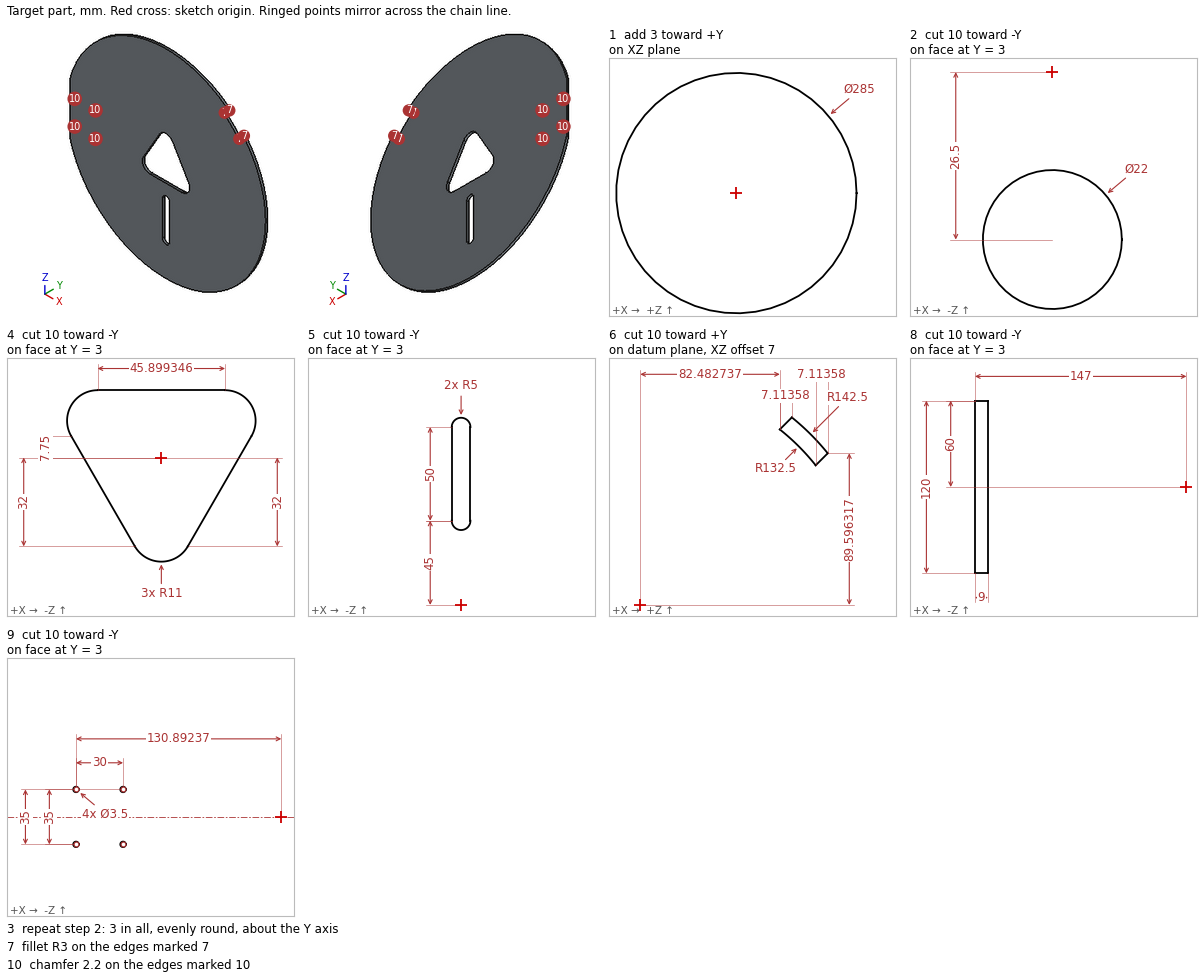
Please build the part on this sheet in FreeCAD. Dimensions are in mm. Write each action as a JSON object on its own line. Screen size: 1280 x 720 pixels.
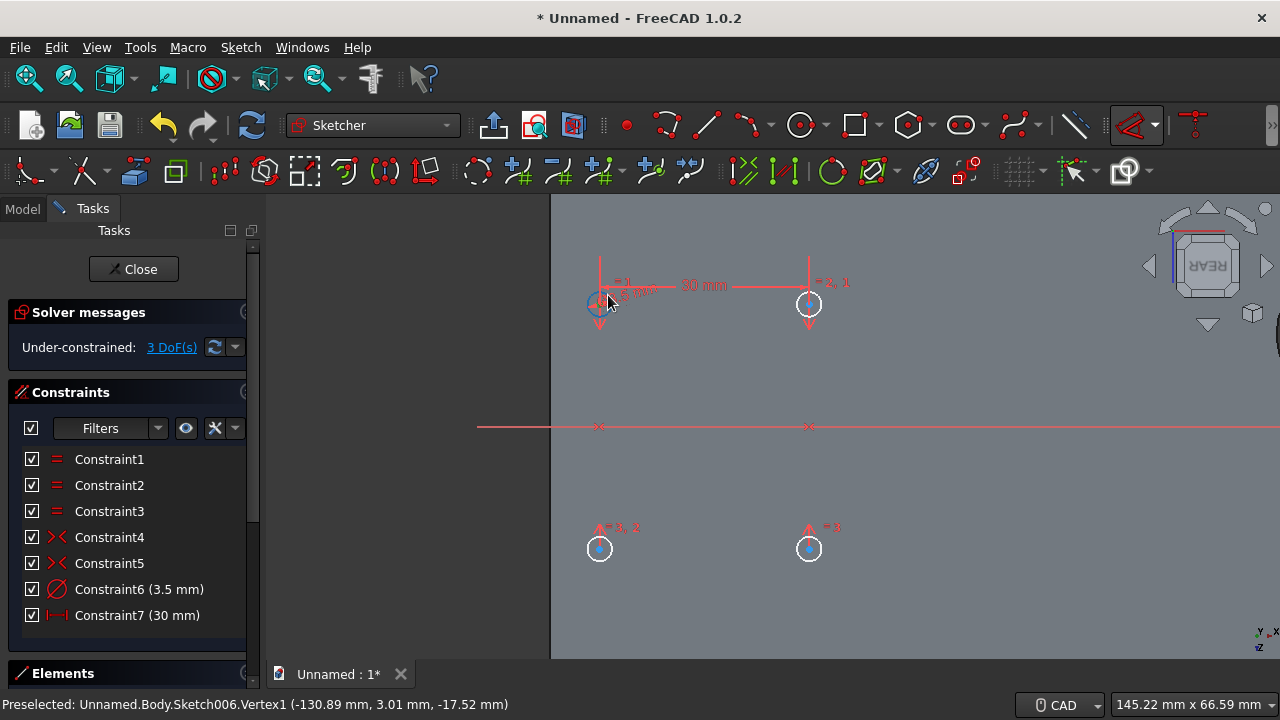
{"action": "left_click", "coordinate": [600, 549]}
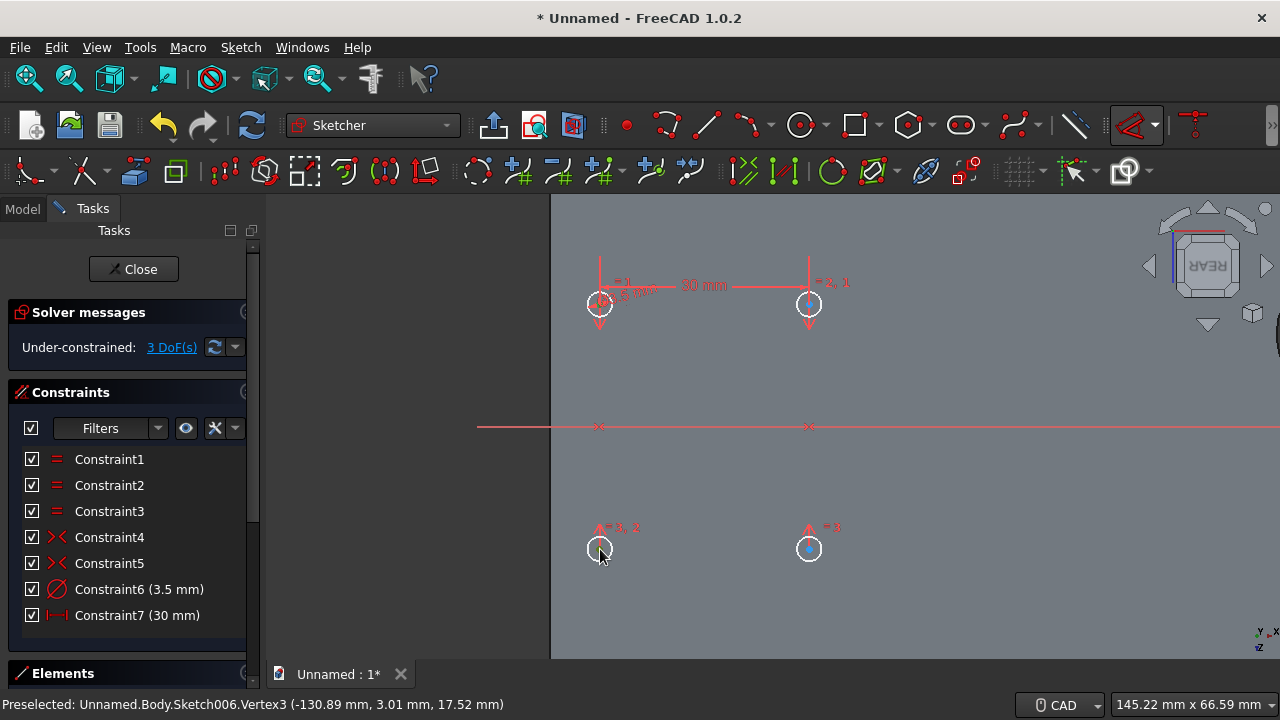
{"action": "key", "text": "i"}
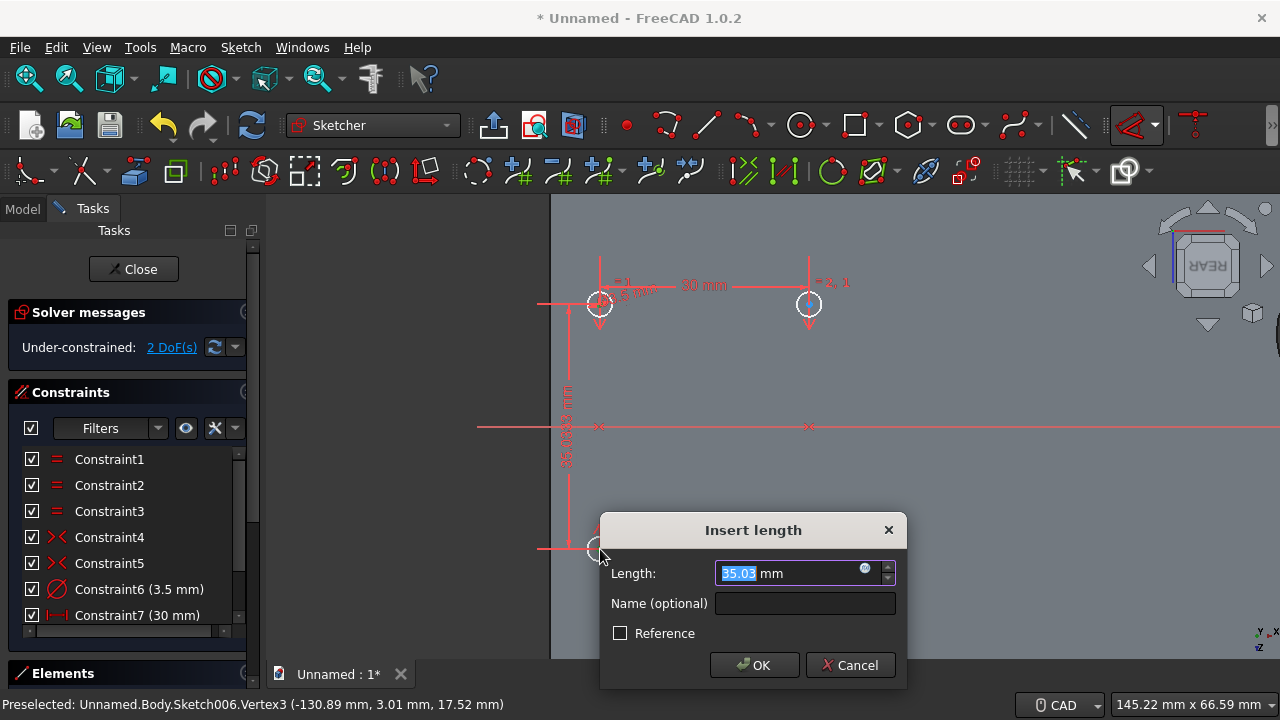
{"action": "type", "text": "35"}
{"action": "key", "text": "Return"}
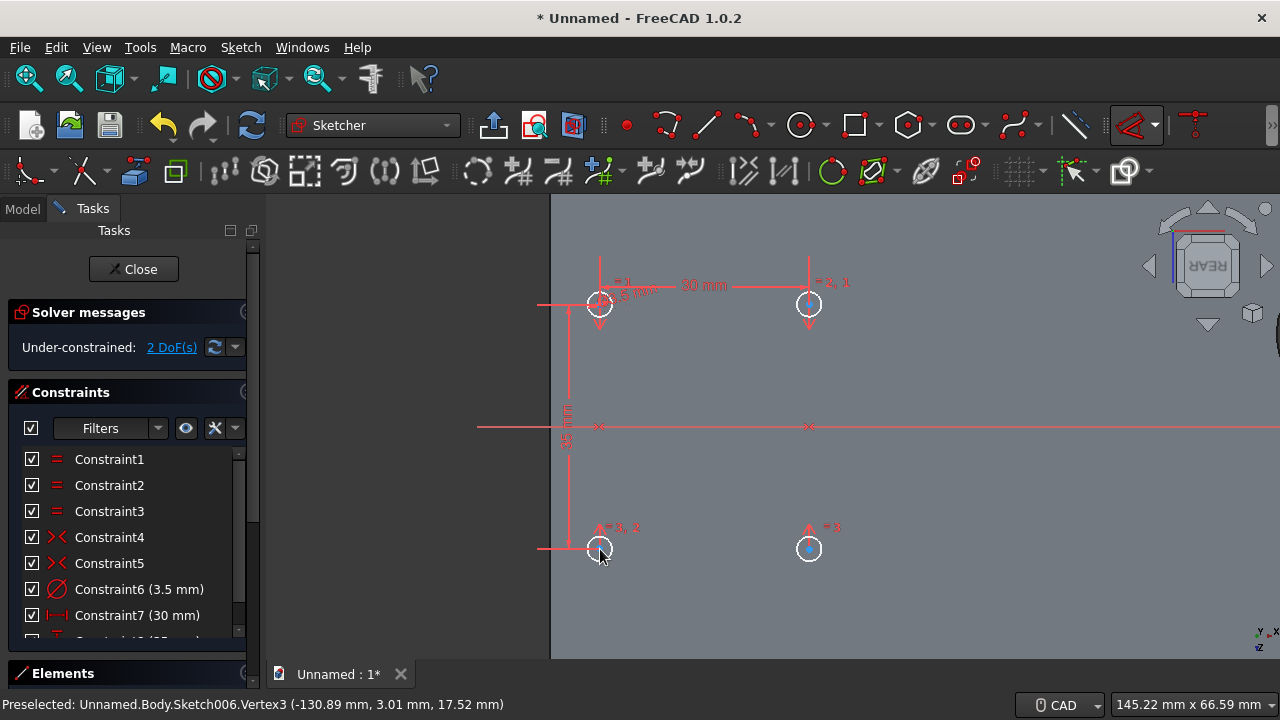
{"action": "left_click", "coordinate": [809, 304]}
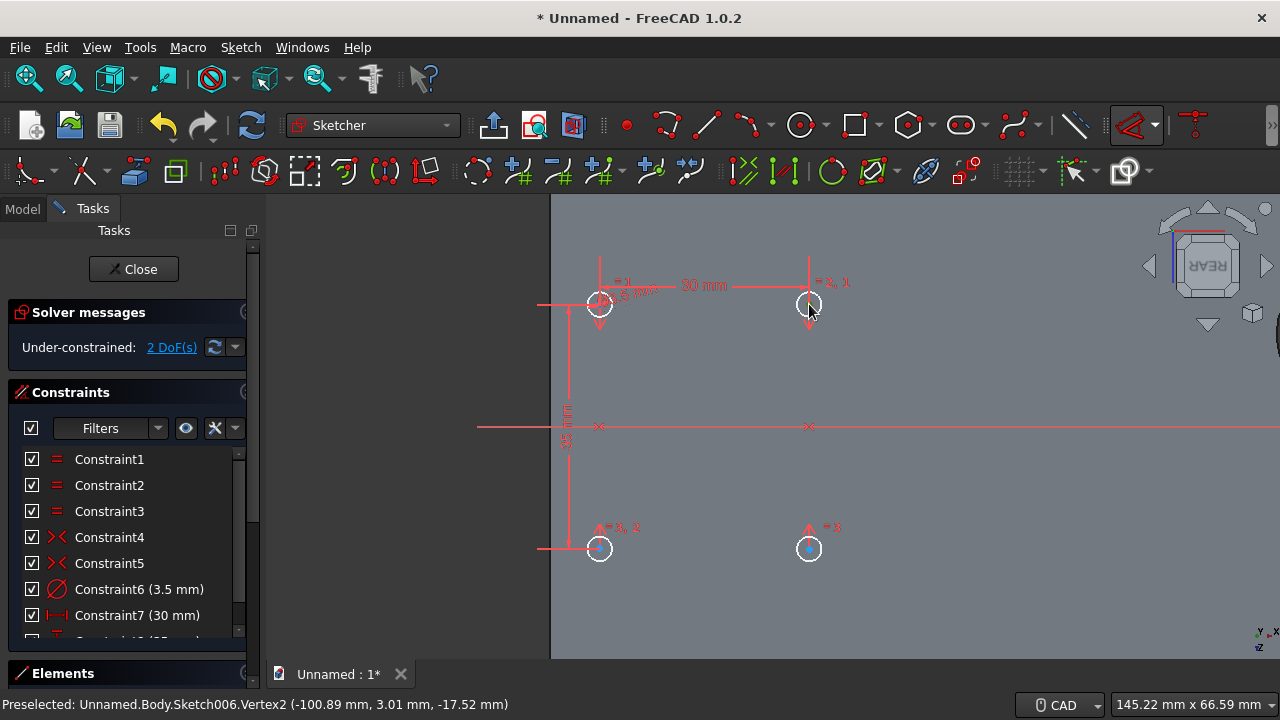
{"action": "left_click", "coordinate": [600, 549]}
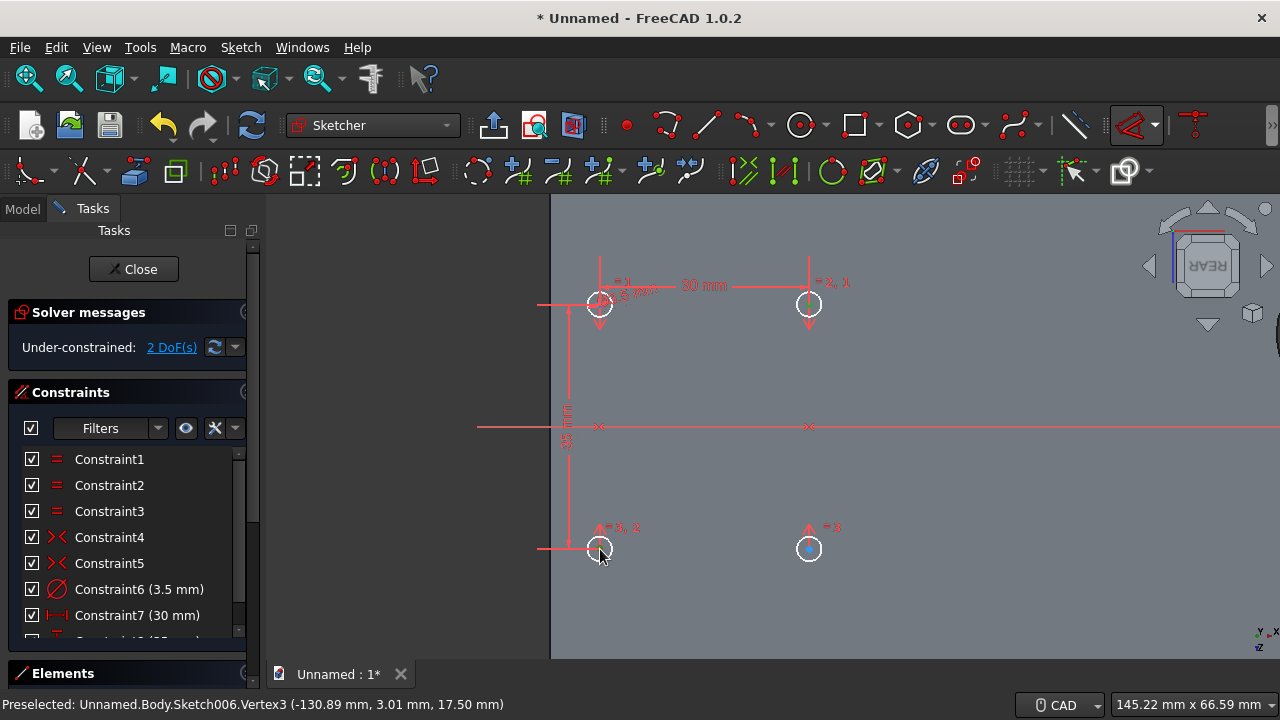
{"action": "key", "text": "i"}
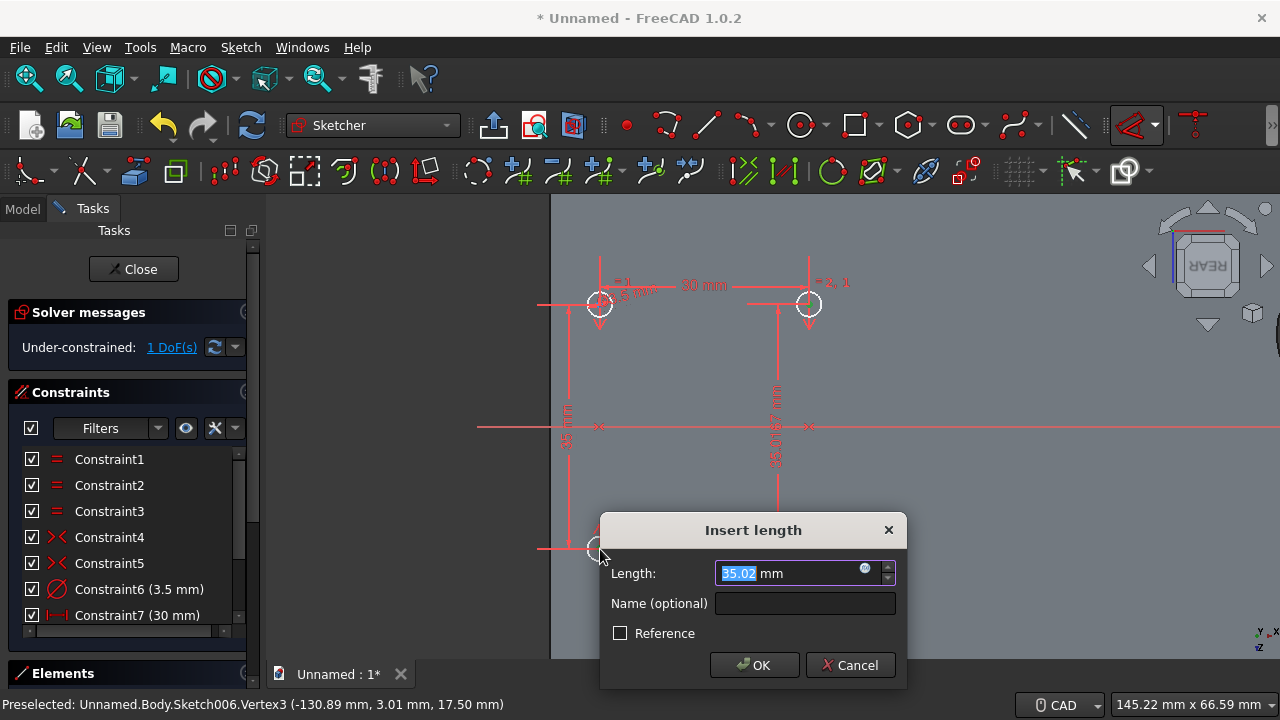
{"action": "type", "text": "35"}
{"action": "key", "text": "Return"}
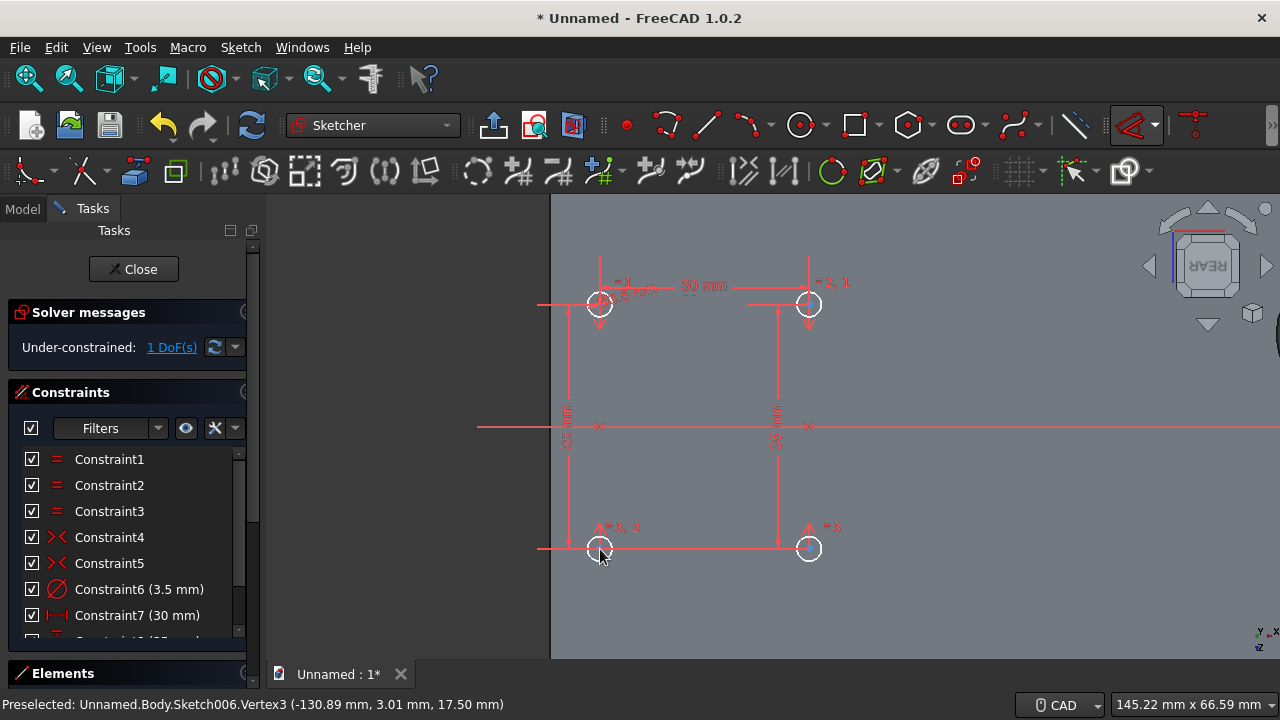
{"action": "left_click", "coordinate": [600, 305]}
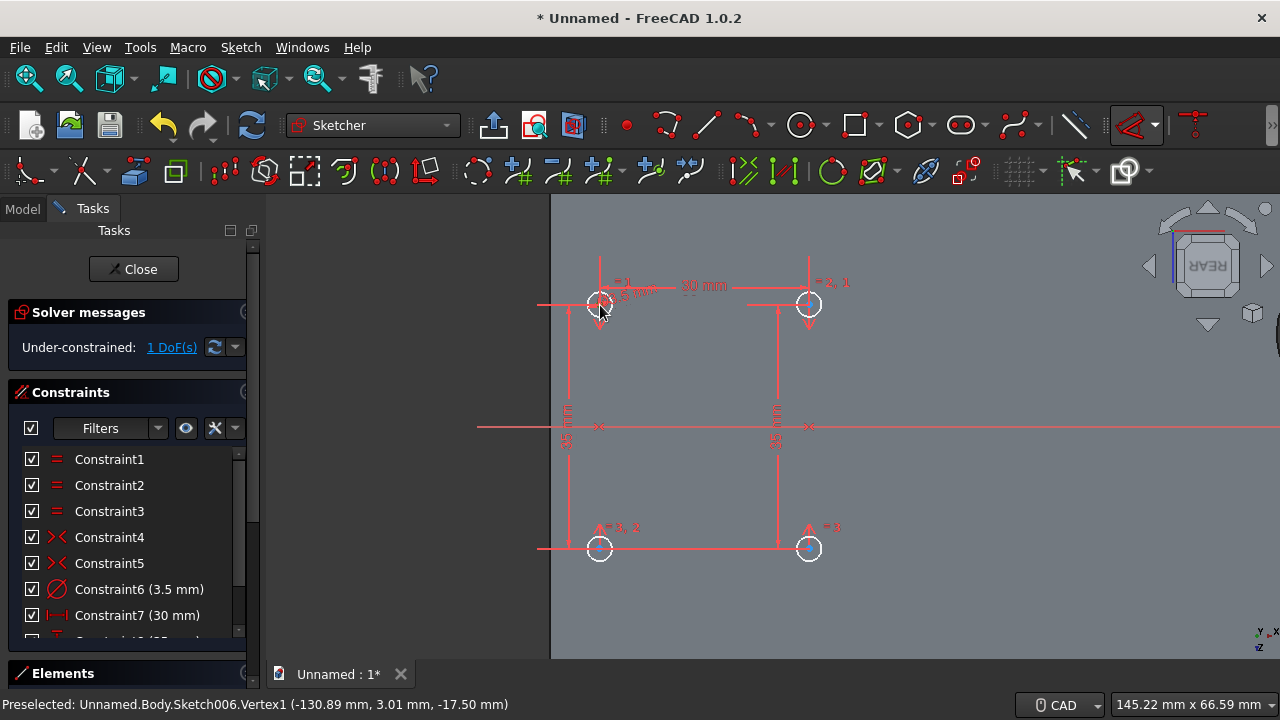
{"action": "left_click", "coordinate": [1158, 126]}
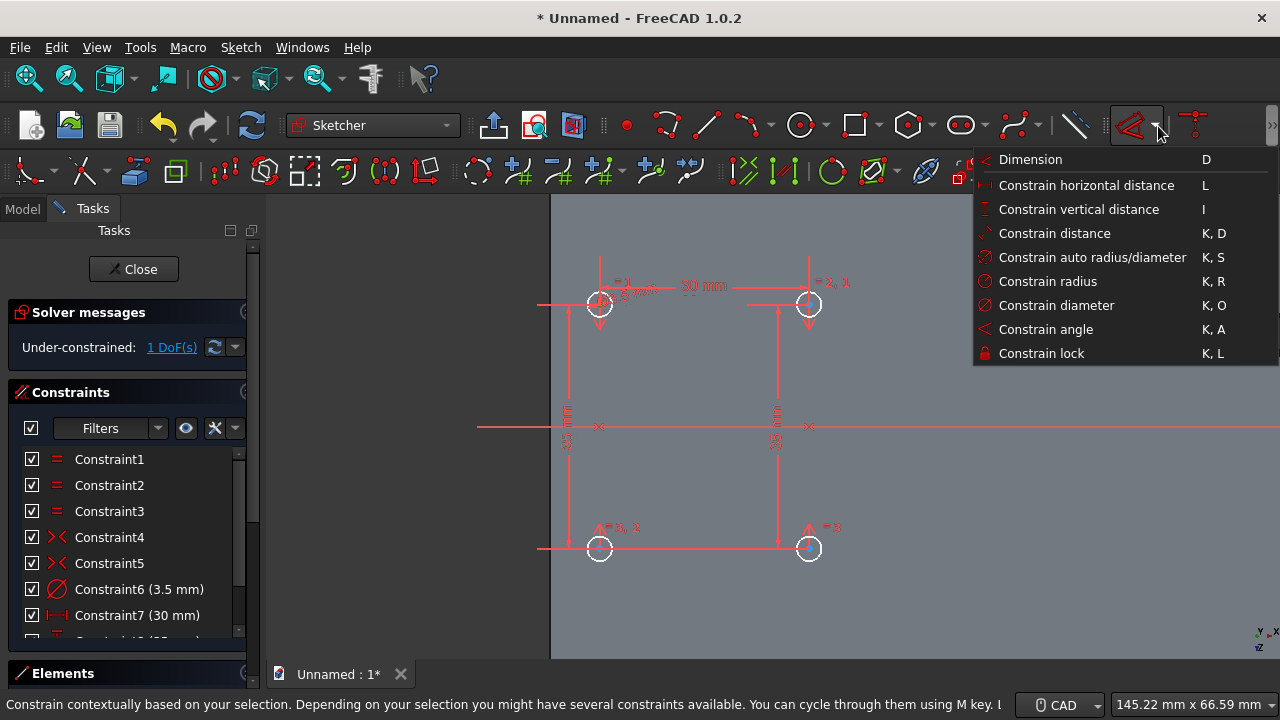
{"action": "left_click", "coordinate": [1126, 185]}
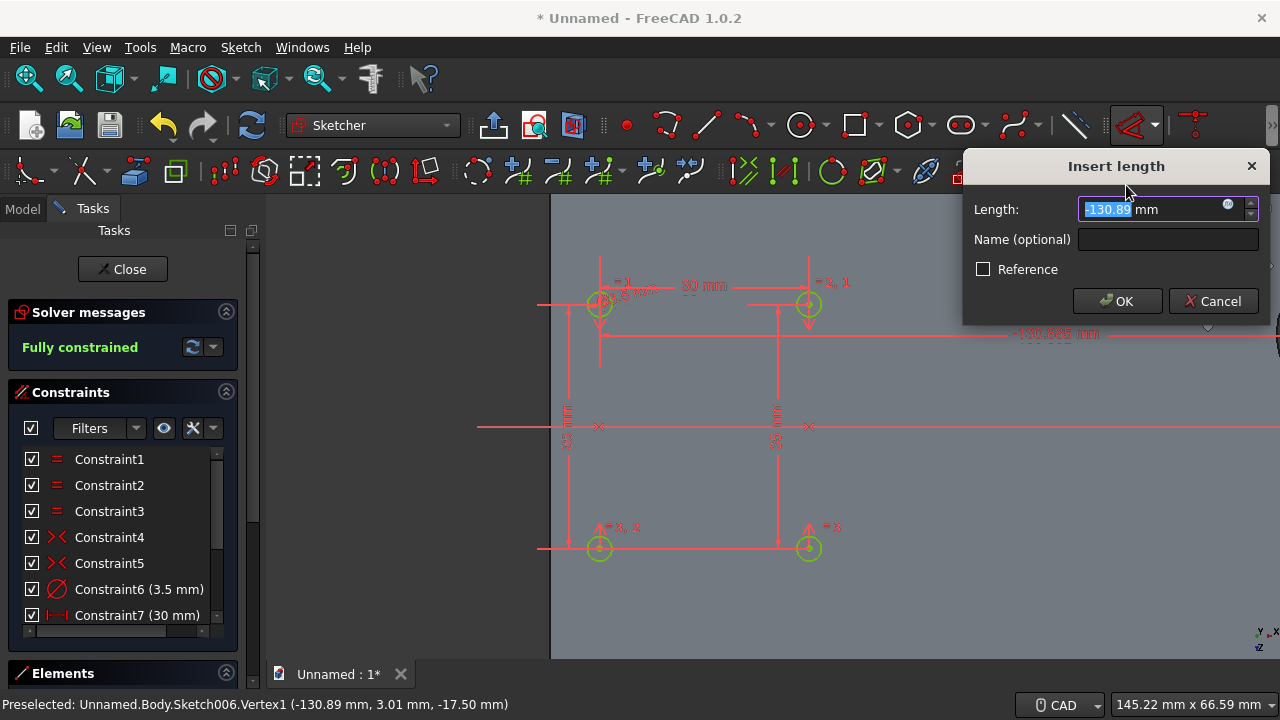
{"action": "type", "text": "-130.89237"}
{"action": "key", "text": "Return"}